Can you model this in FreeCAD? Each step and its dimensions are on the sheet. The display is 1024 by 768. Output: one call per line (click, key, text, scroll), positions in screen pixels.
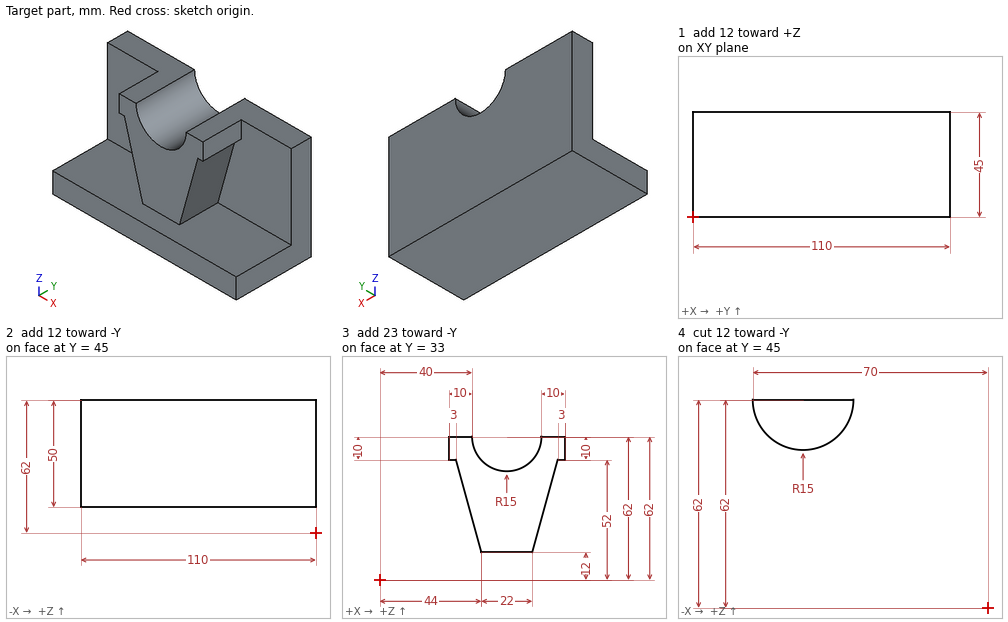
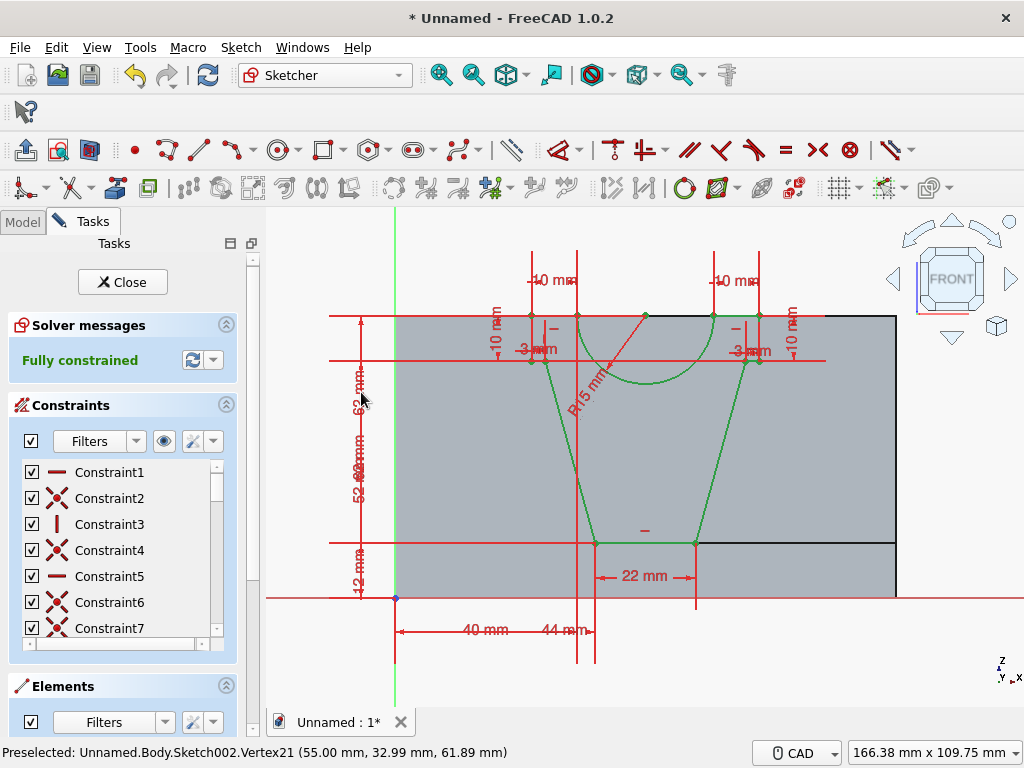
click(123, 282)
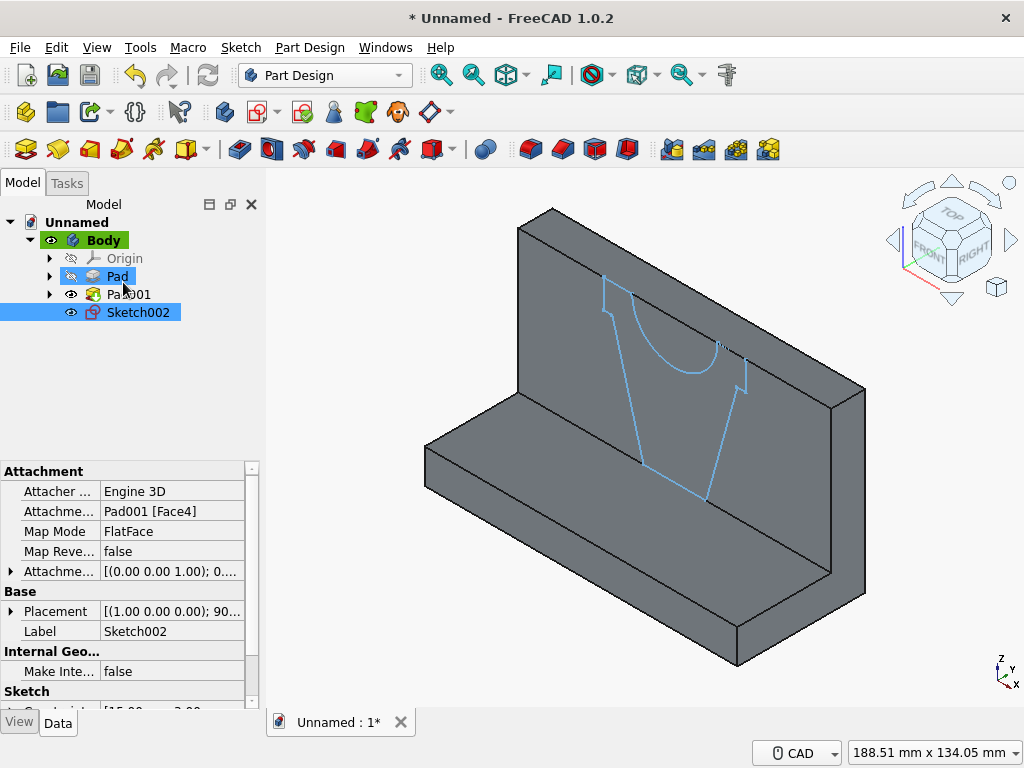
click(26, 150)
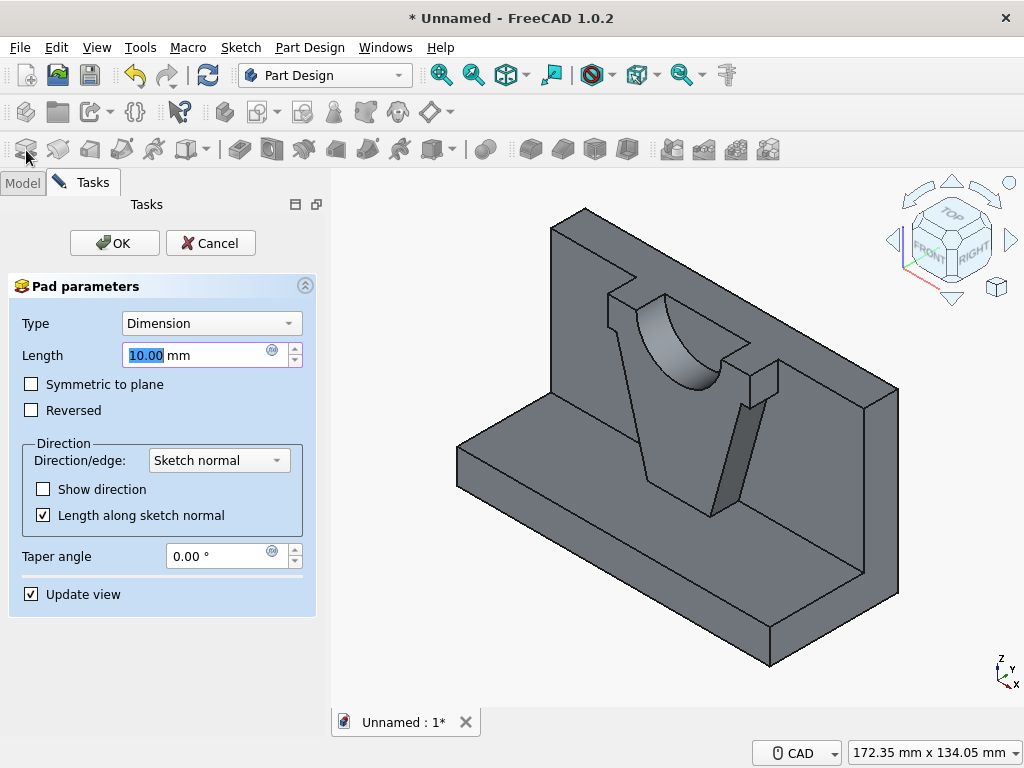
text(23)
key(Tab)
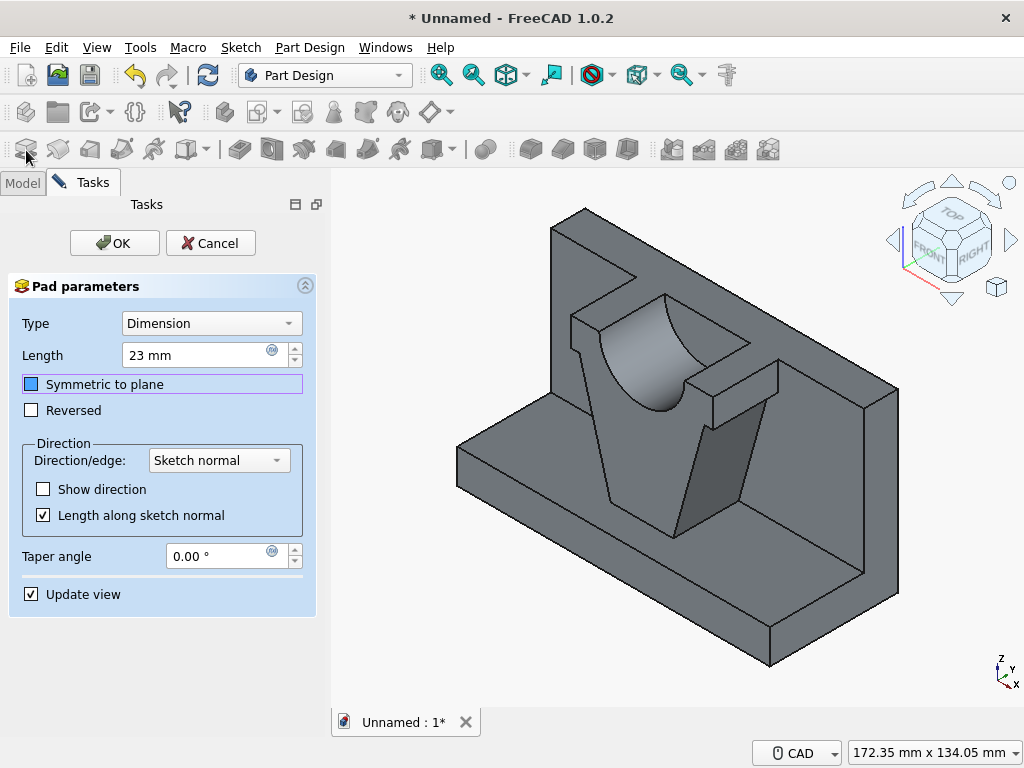
click(115, 243)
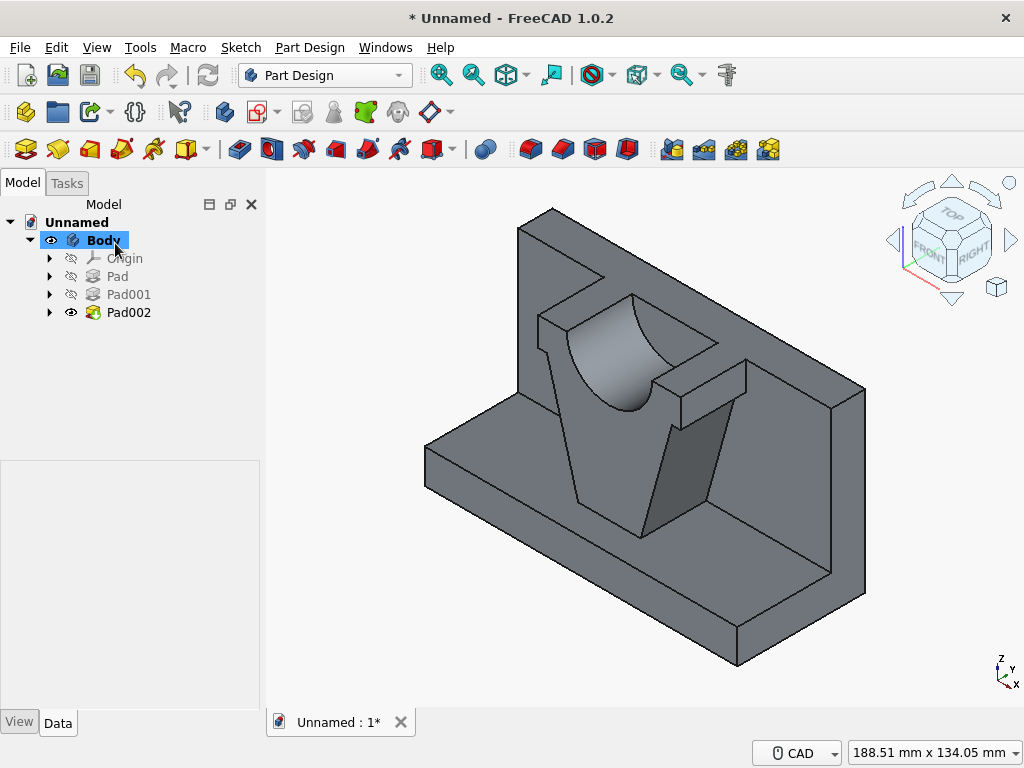
key(4)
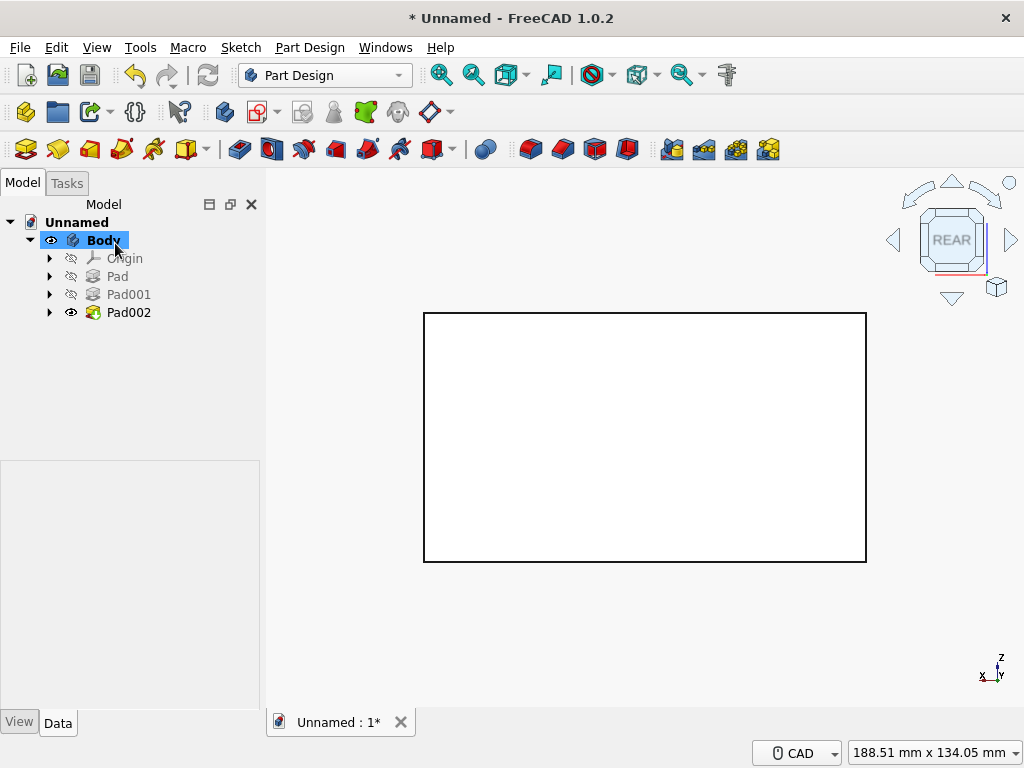
click(582, 436)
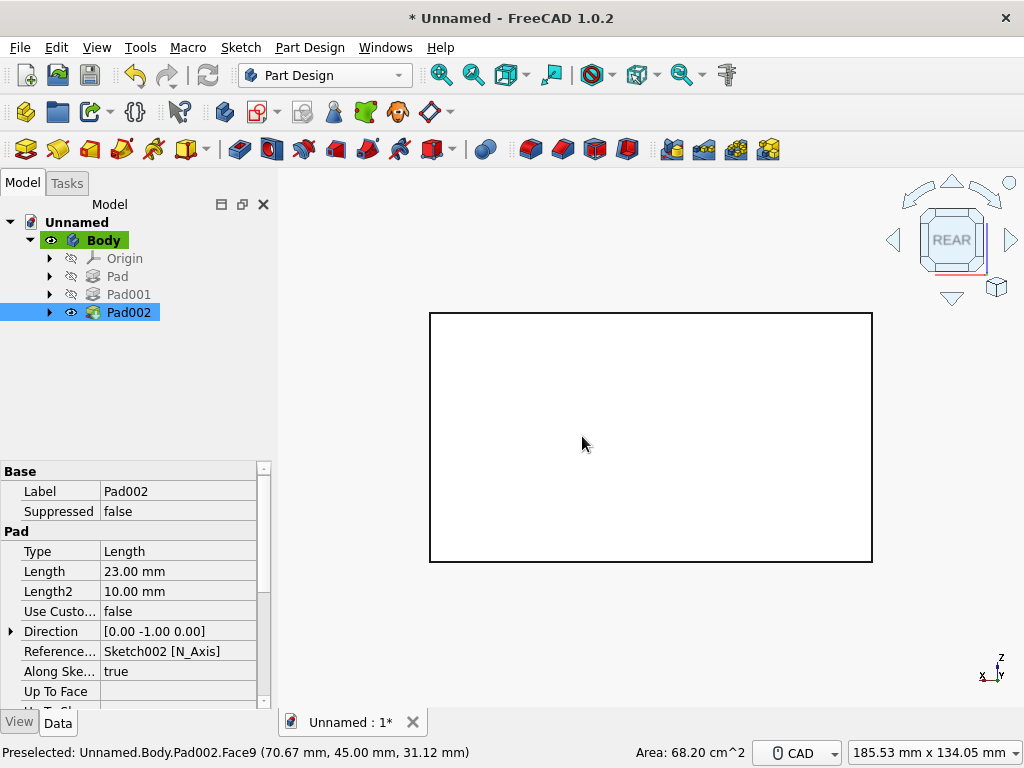
click(258, 112)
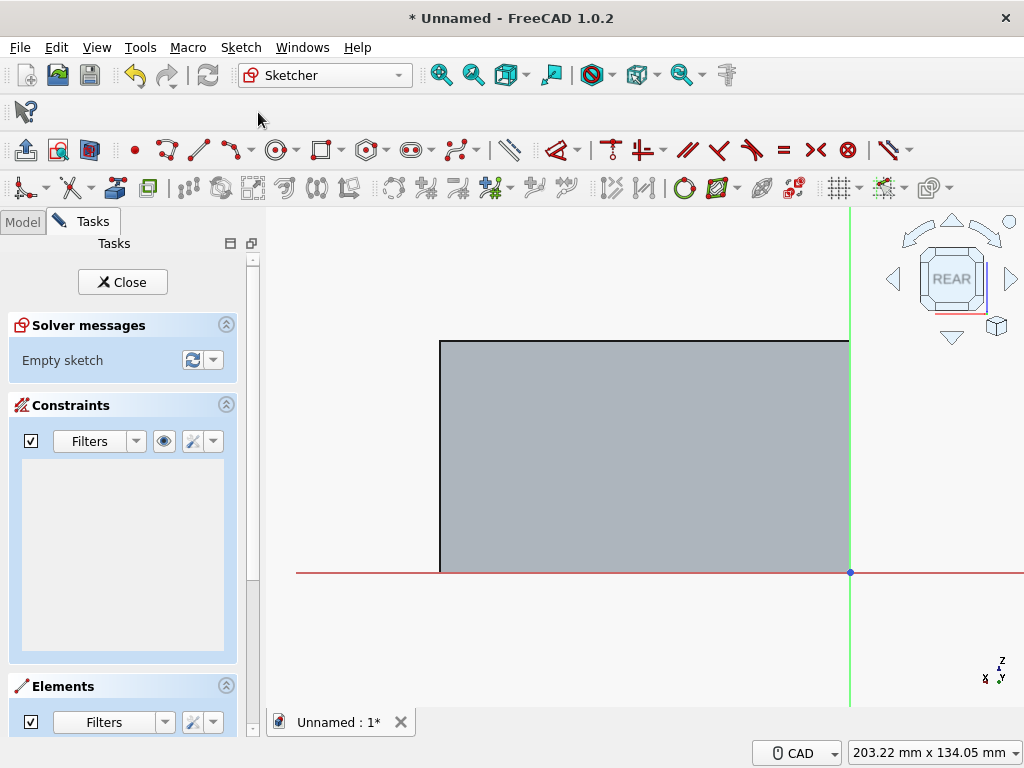
scroll(294, 457, down, 1)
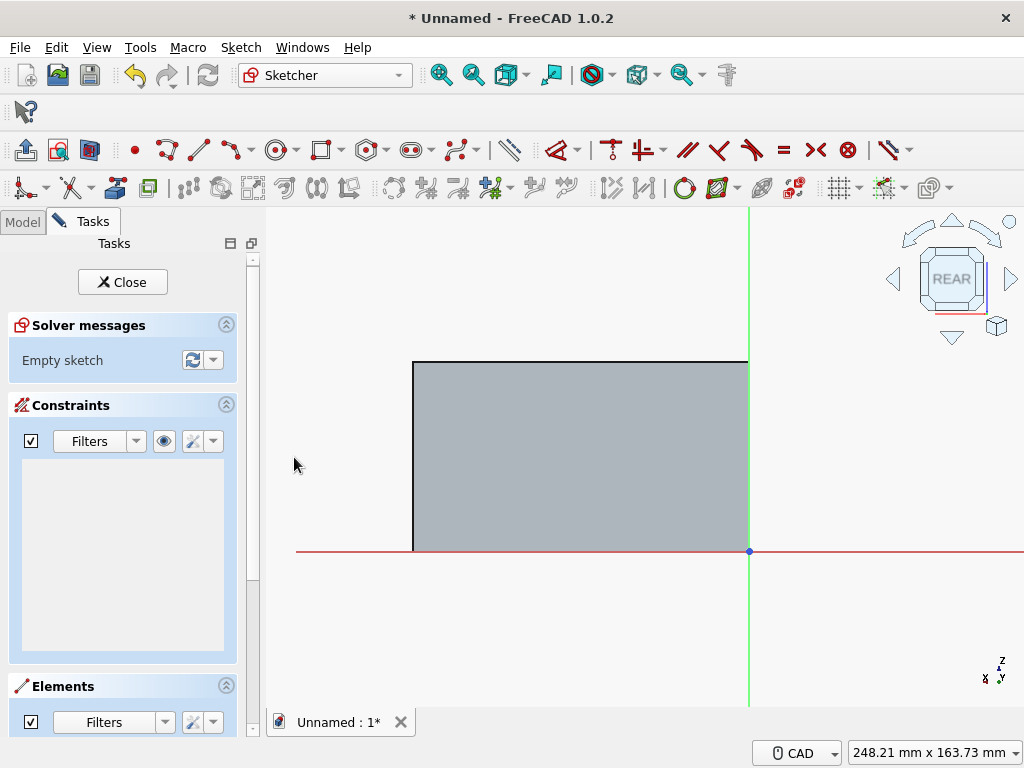
scroll(723, 457, up, 3)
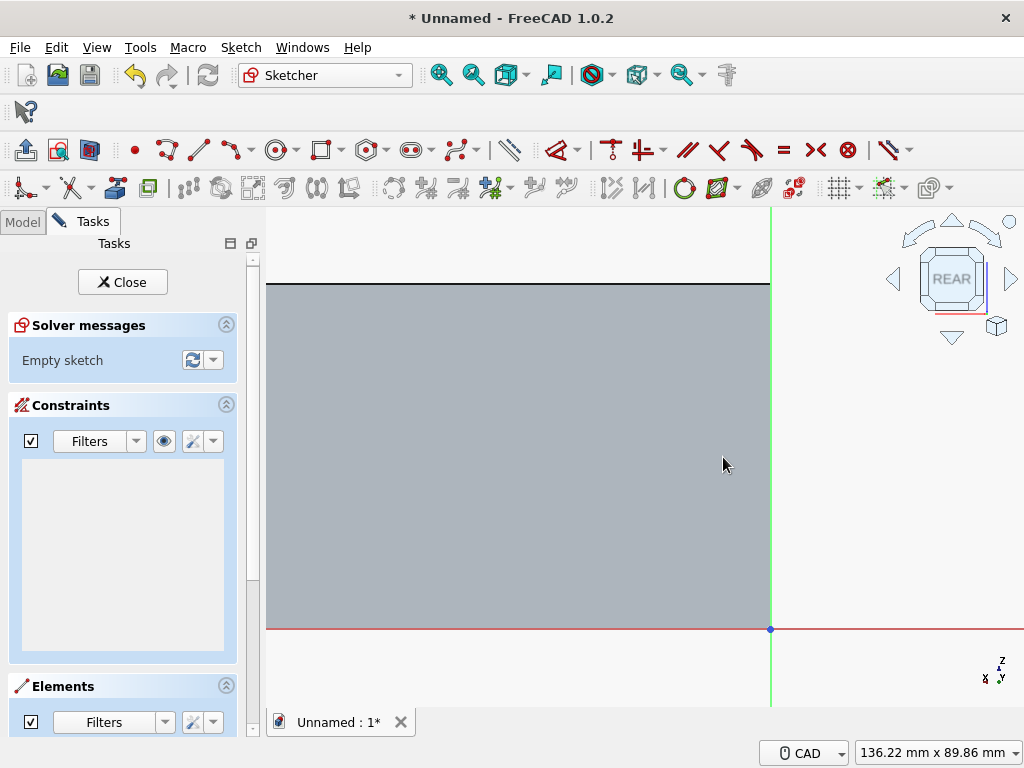
click(200, 150)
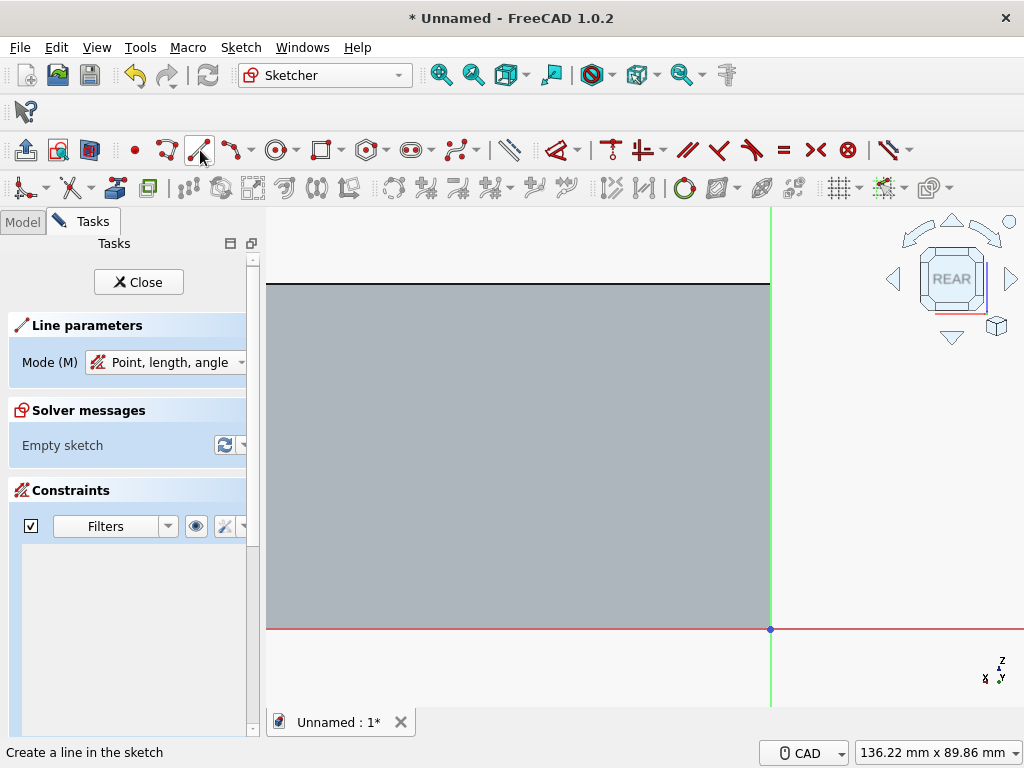
click(381, 284)
click(548, 284)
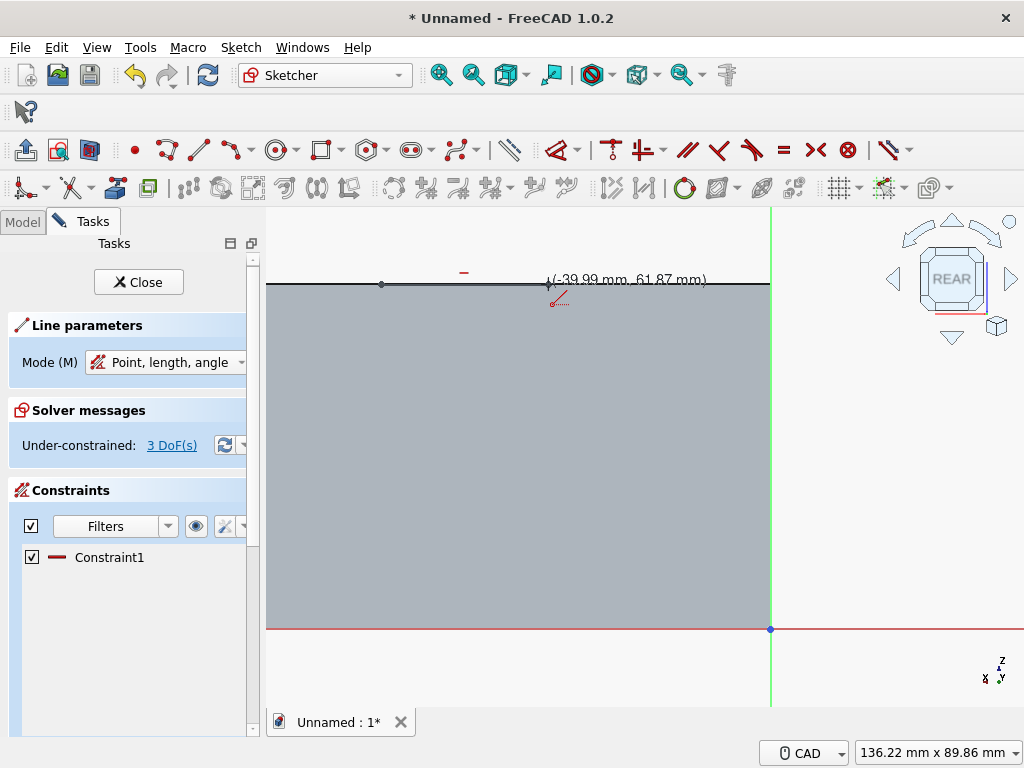
click(232, 150)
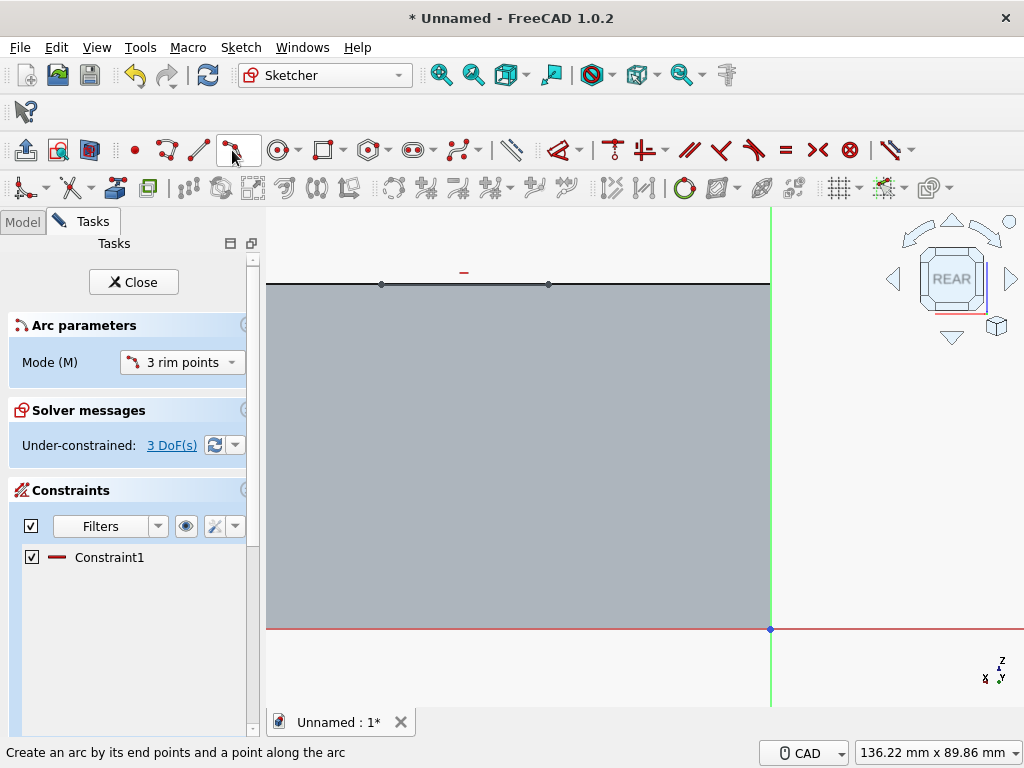
click(548, 285)
click(381, 285)
click(464, 368)
key(Escape)